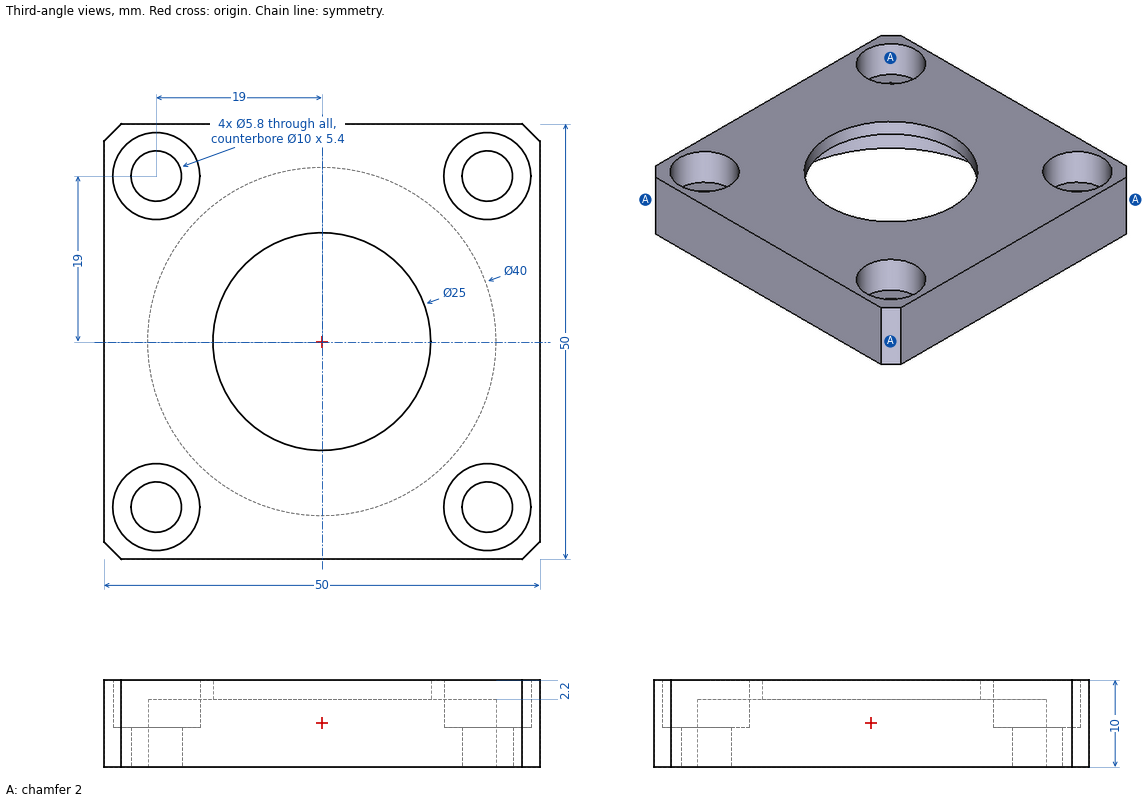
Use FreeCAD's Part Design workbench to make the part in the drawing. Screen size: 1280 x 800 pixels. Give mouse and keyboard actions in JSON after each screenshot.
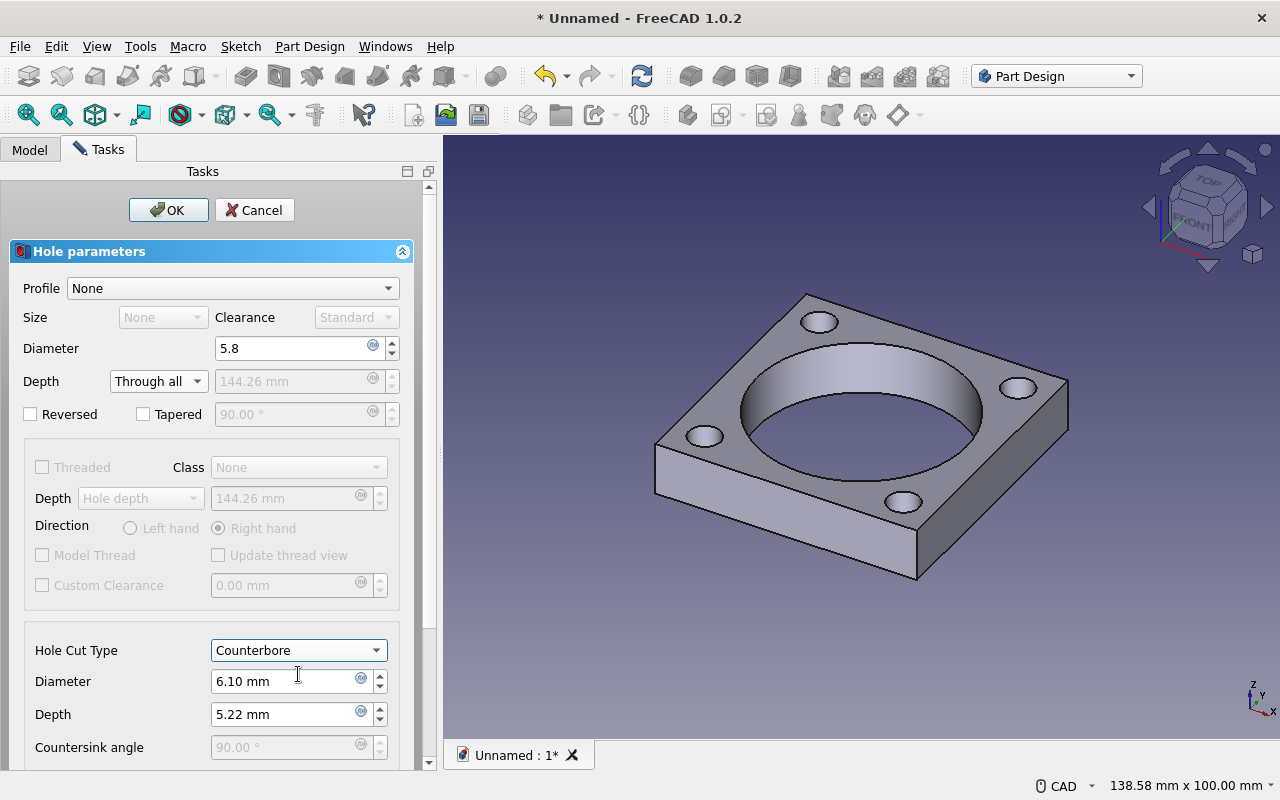
{"action": "triple_click", "coordinate": [292, 682]}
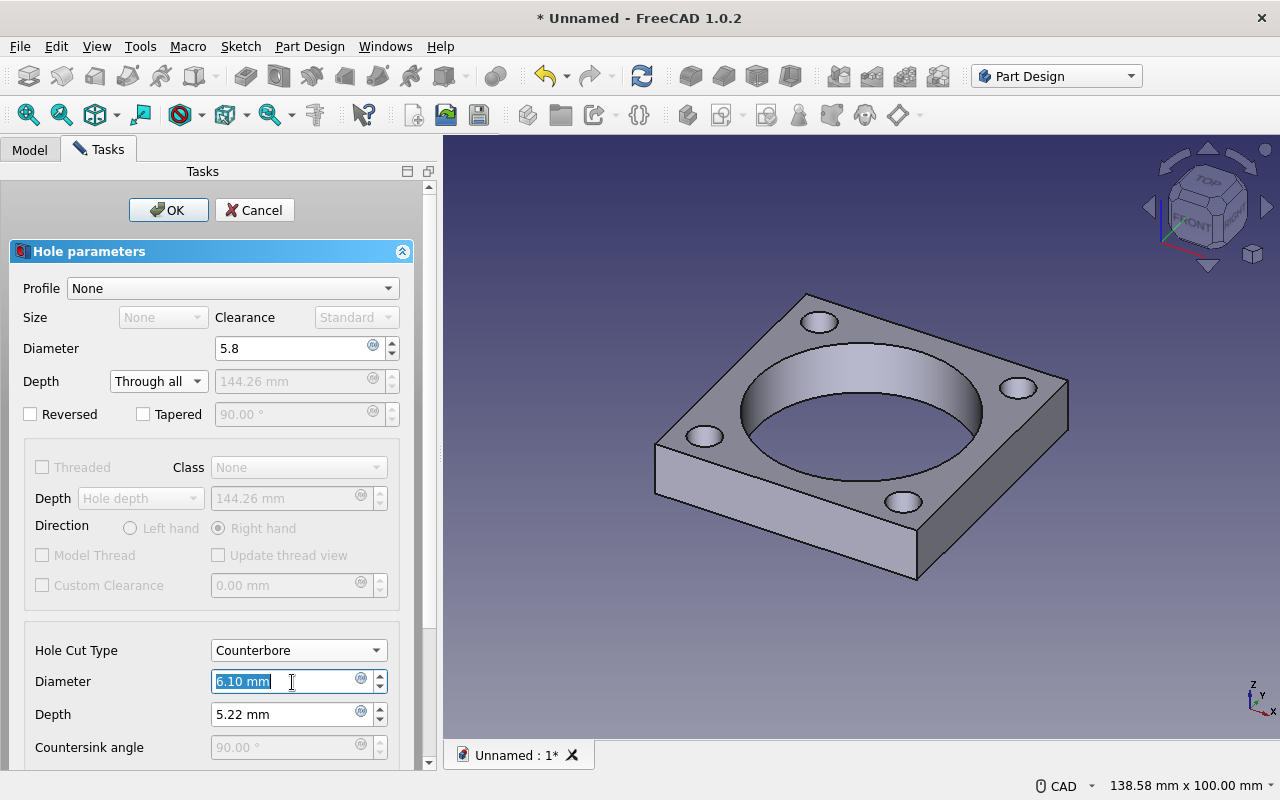
{"action": "type", "text": "10"}
{"action": "key", "text": "Tab"}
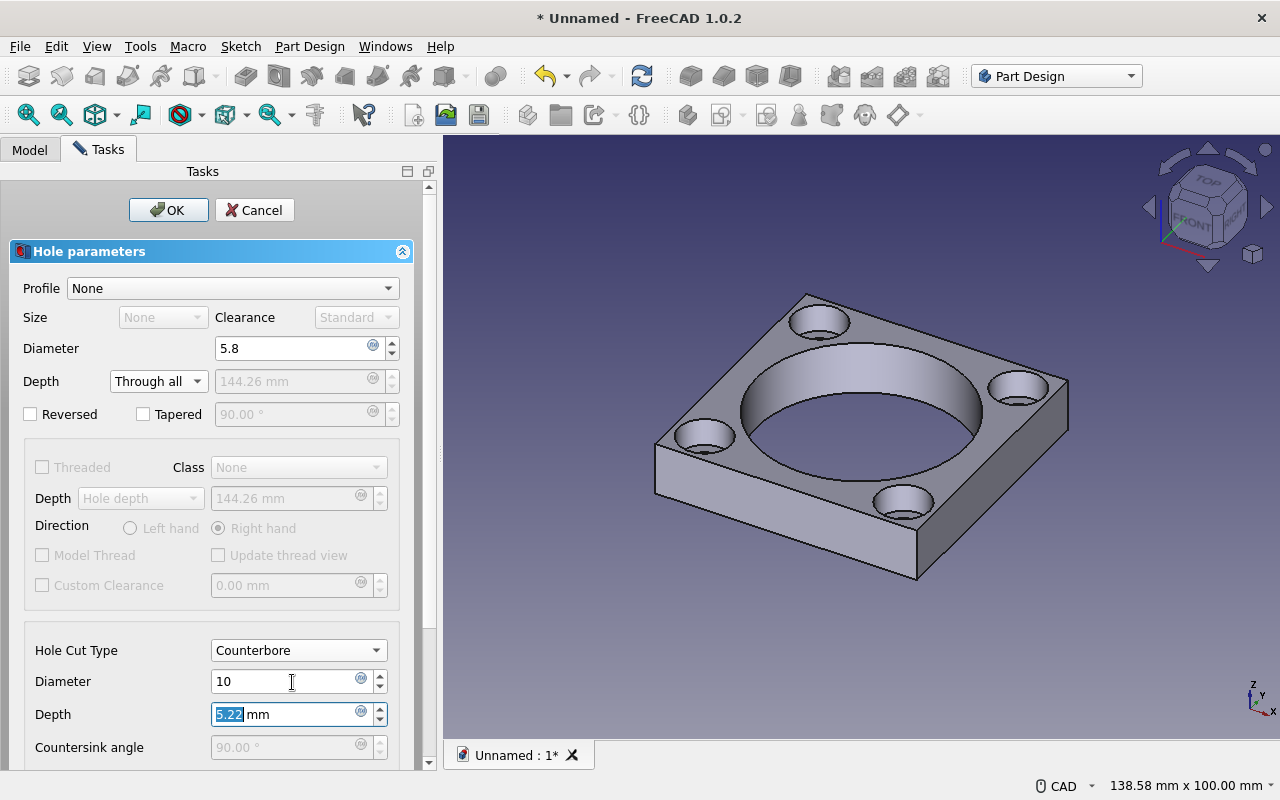
{"action": "type", "text": "5.4"}
{"action": "key", "text": "Tab"}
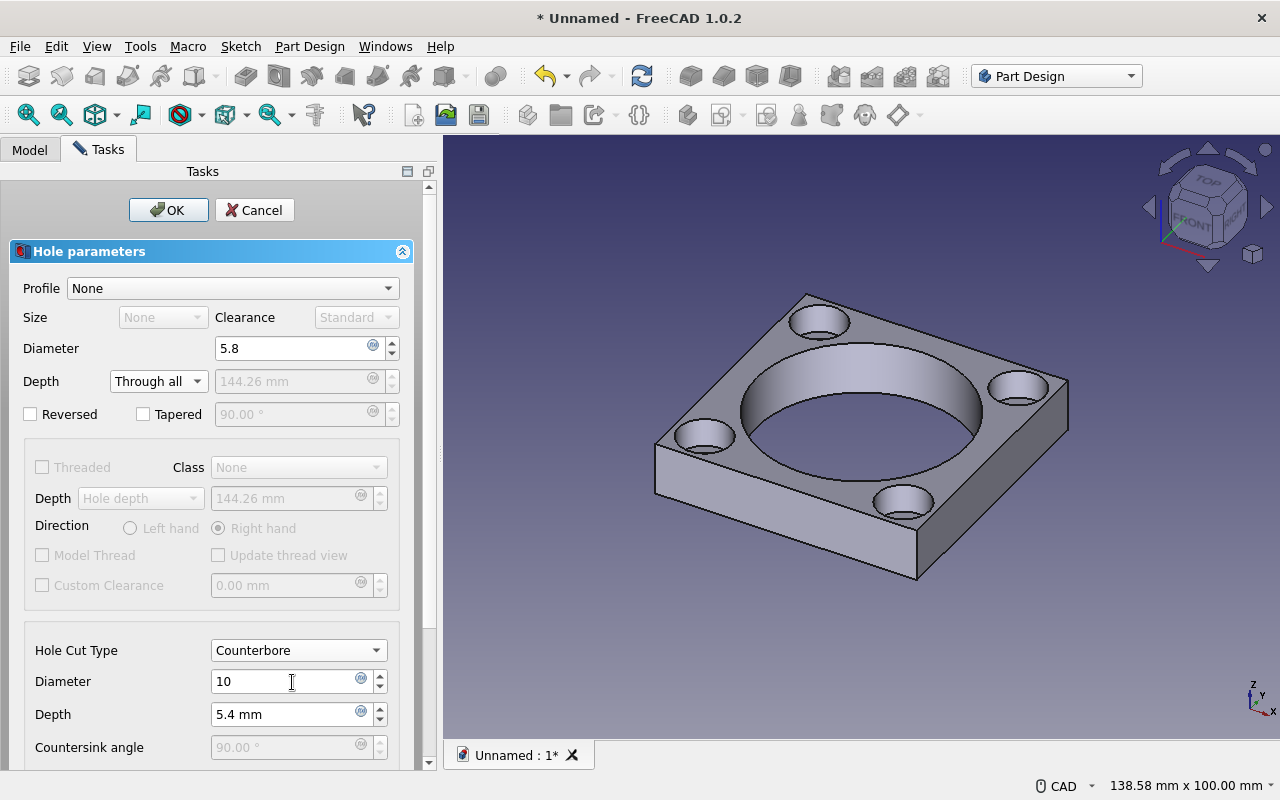
{"action": "left_click", "coordinate": [169, 210]}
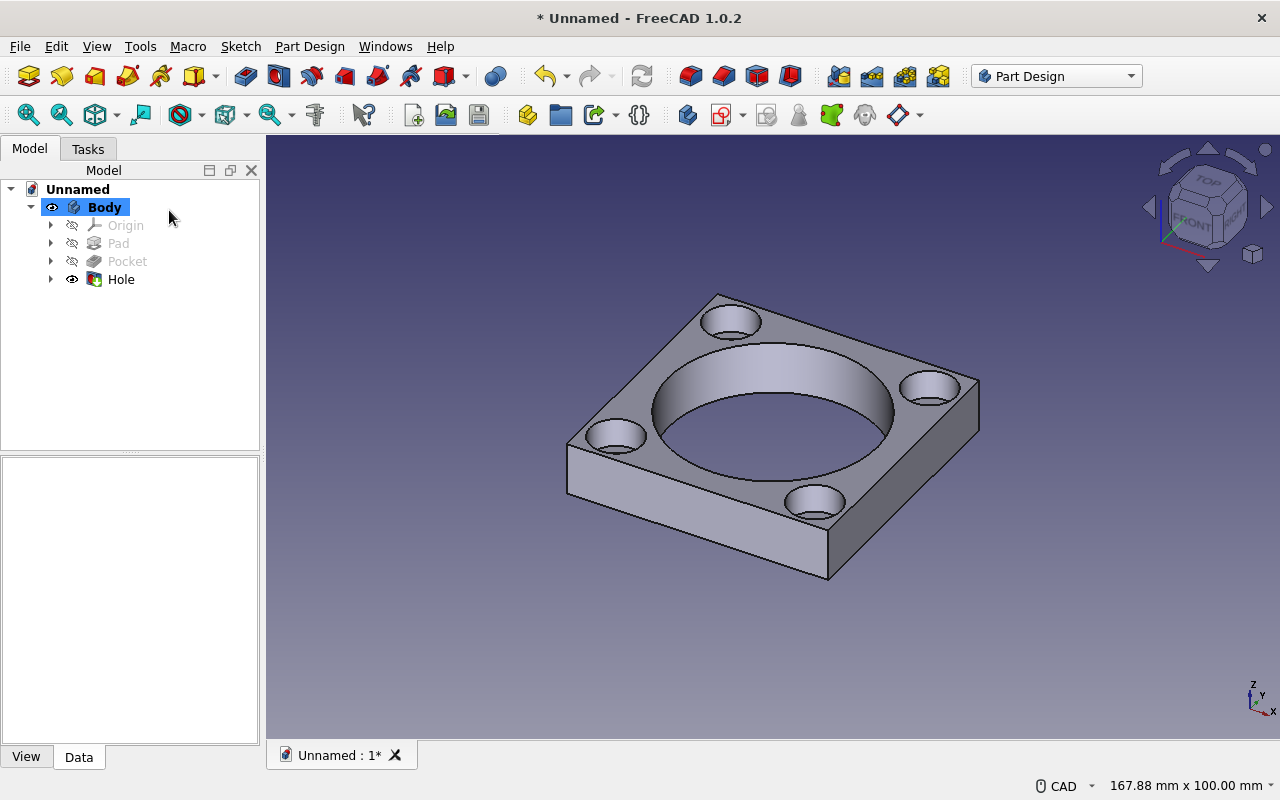
{"action": "left_click", "coordinate": [828, 554]}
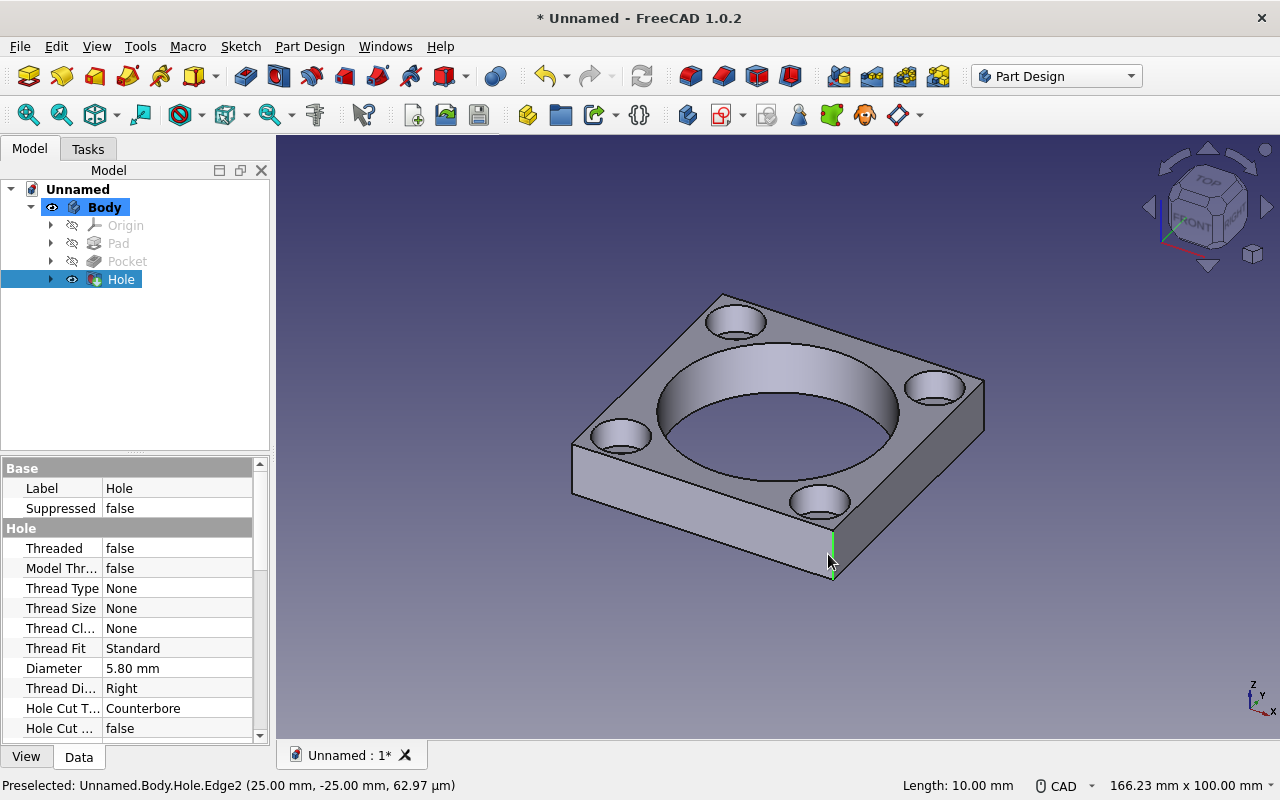
{"action": "key", "text": "0"}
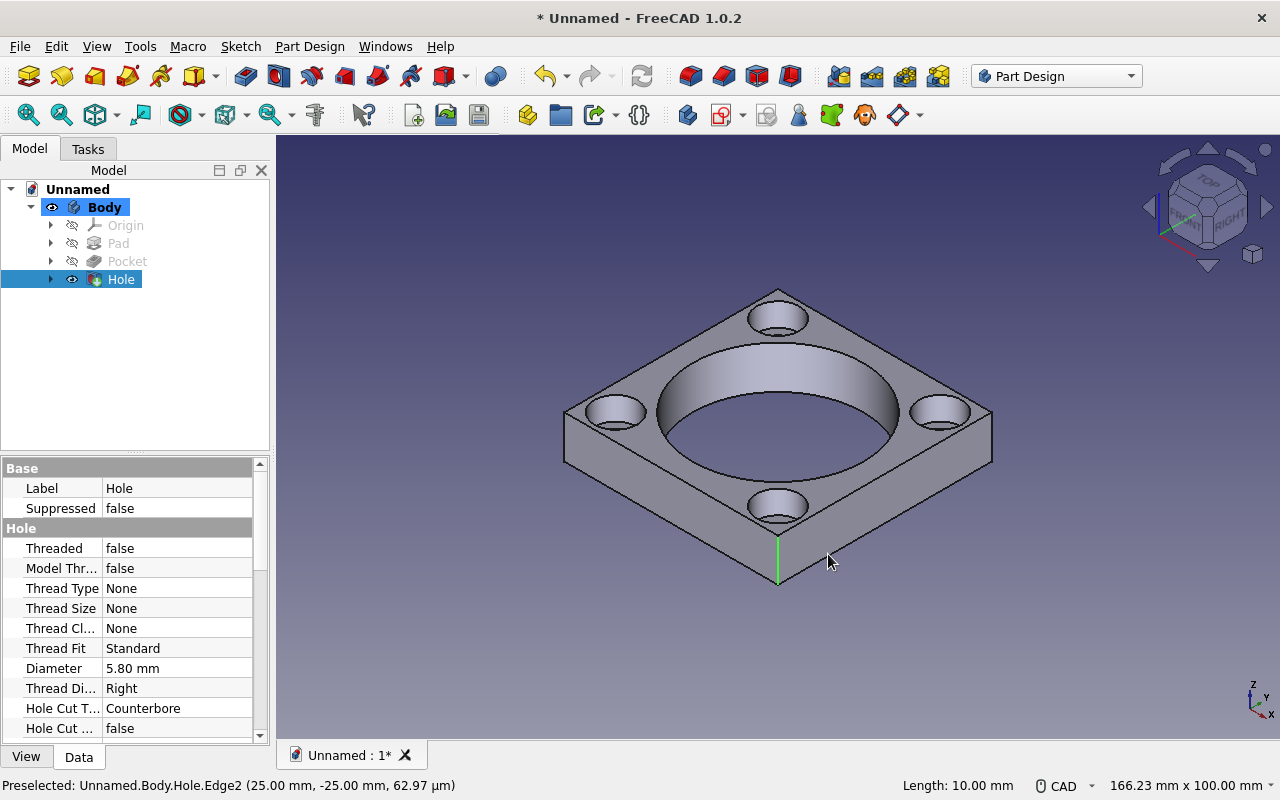
{"action": "key", "text": "2"}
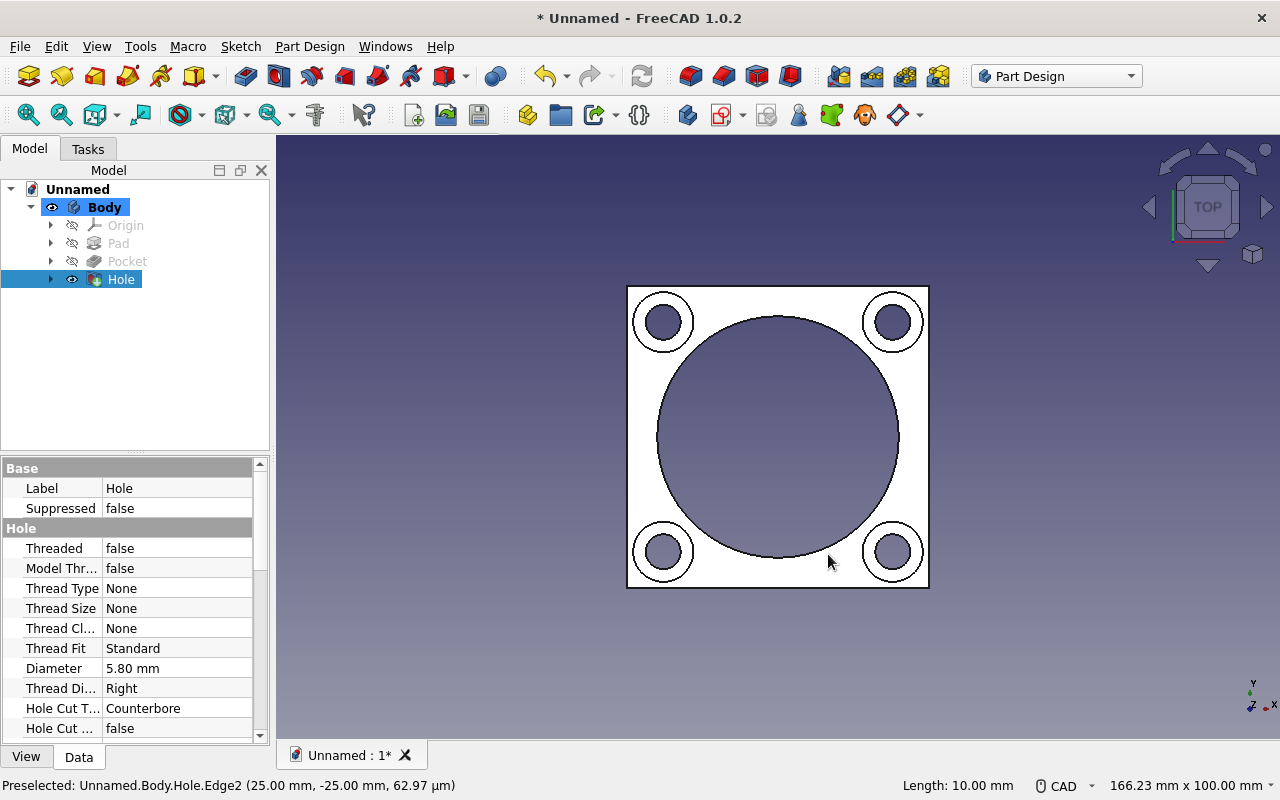
{"action": "key", "text": "1"}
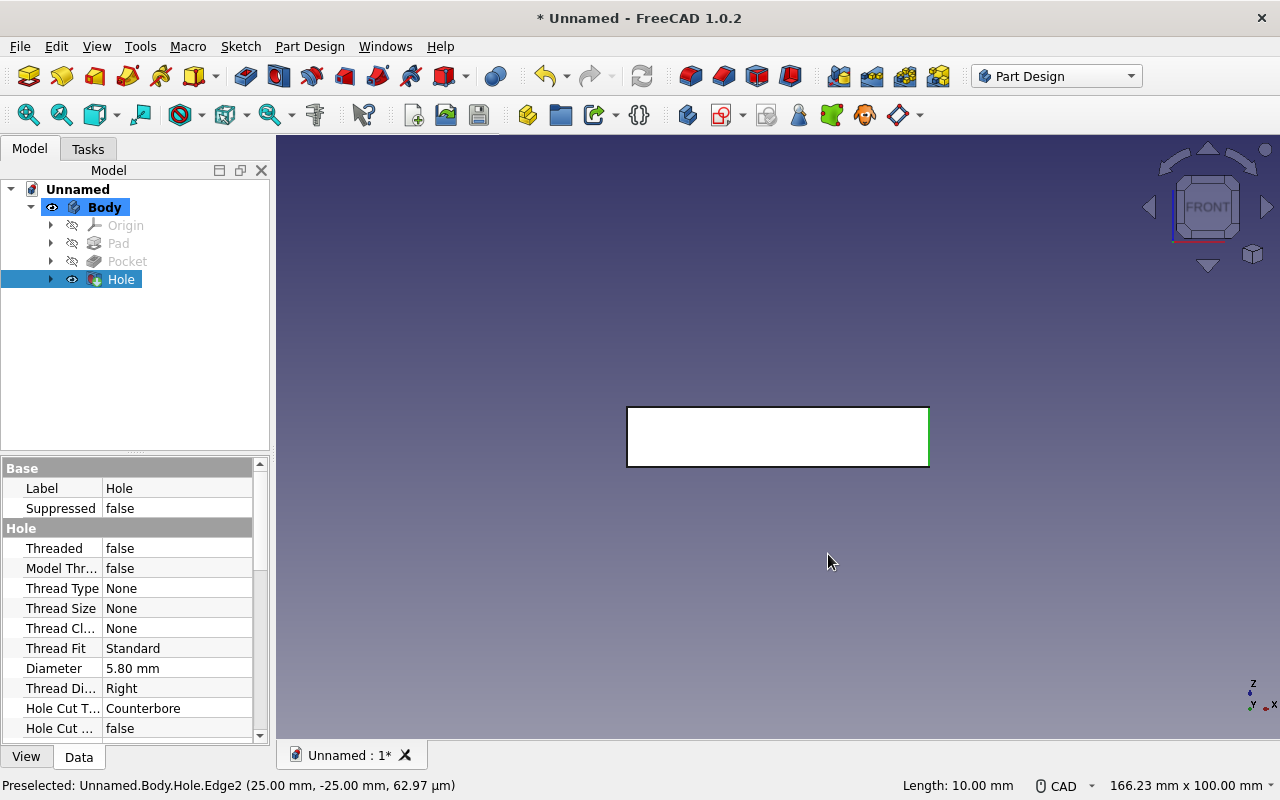
{"action": "left_click", "coordinate": [29, 116]}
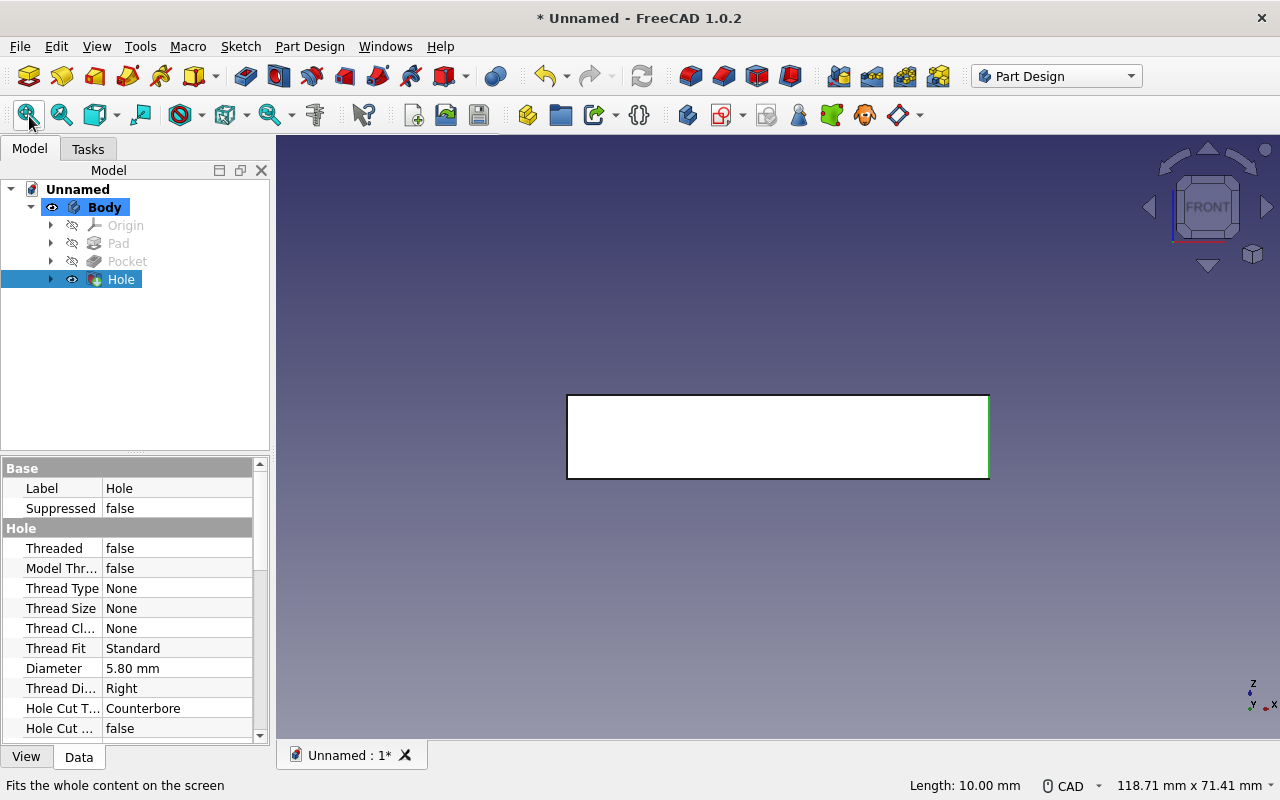
{"action": "left_click", "coordinate": [567, 436], "text": "ctrl"}